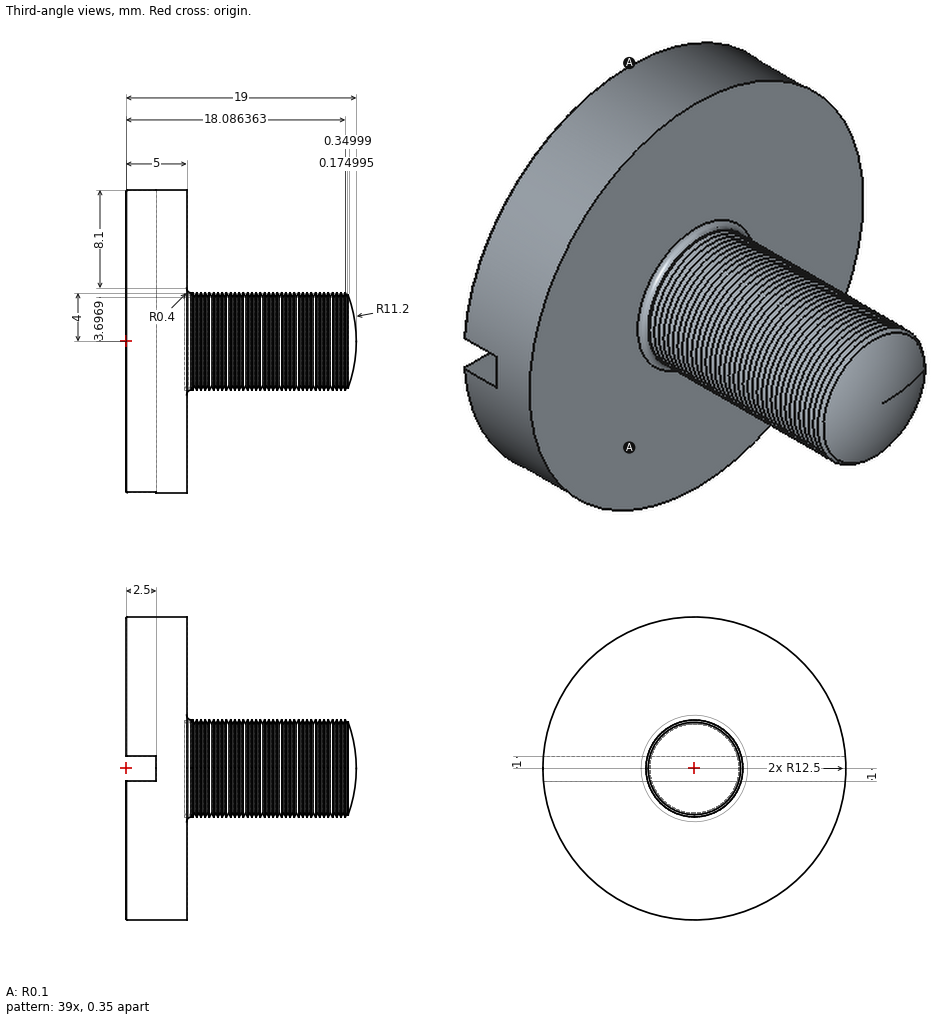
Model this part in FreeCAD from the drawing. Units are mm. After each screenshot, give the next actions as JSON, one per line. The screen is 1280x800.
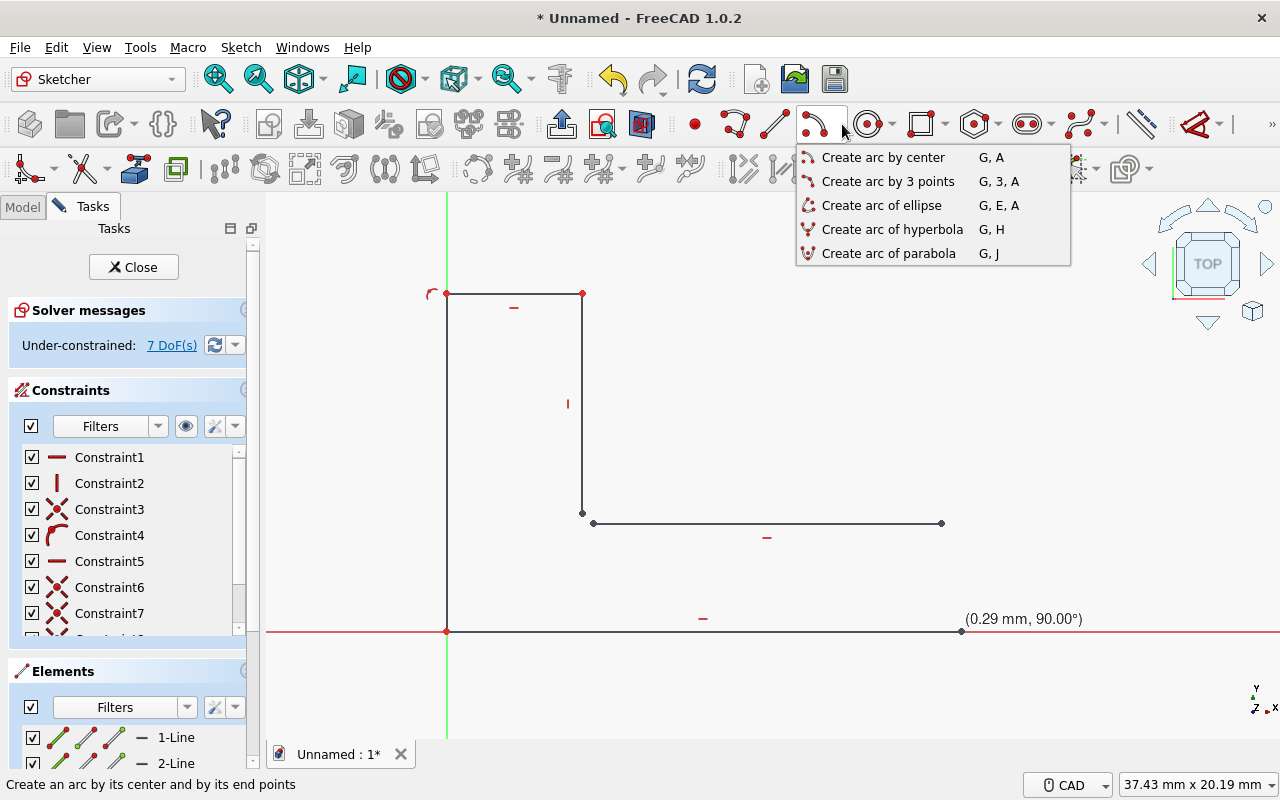
{"action": "left_click", "coordinate": [934, 181]}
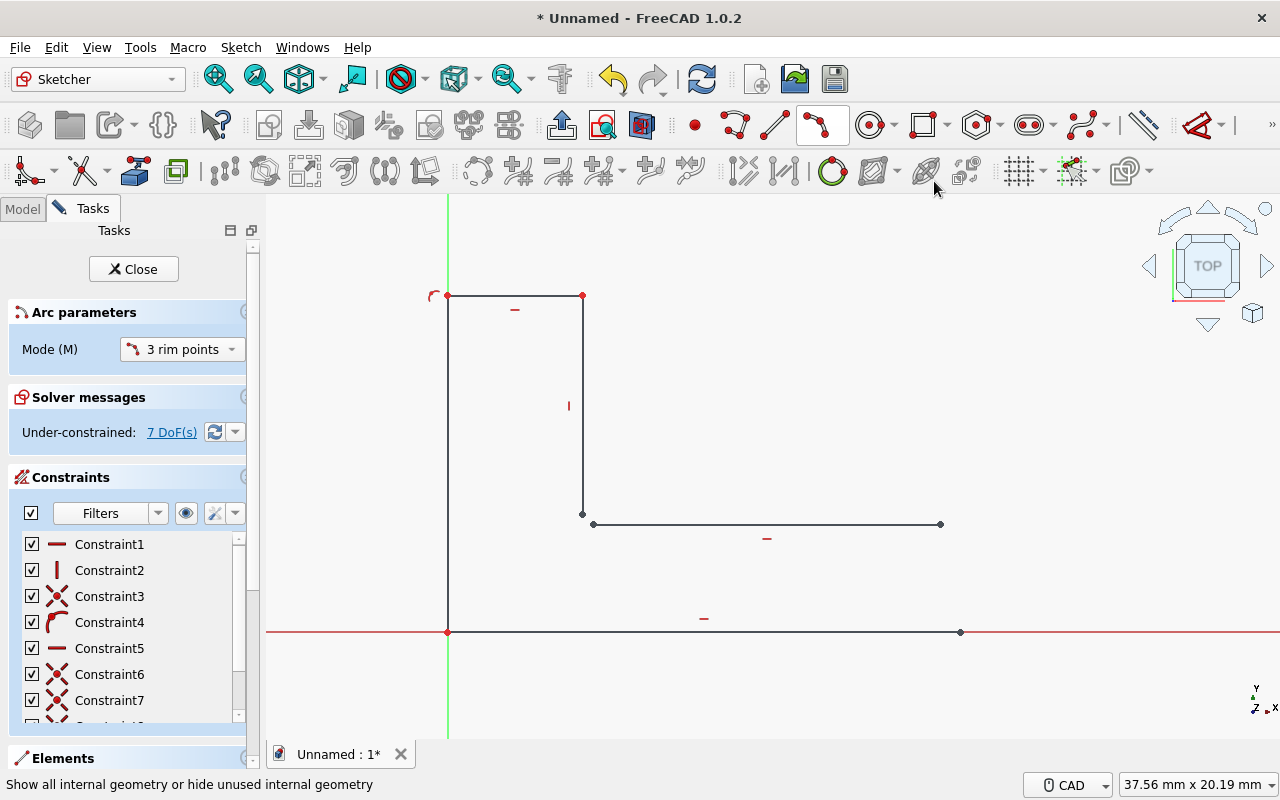
{"action": "left_click", "coordinate": [594, 525]}
{"action": "left_click", "coordinate": [583, 515]}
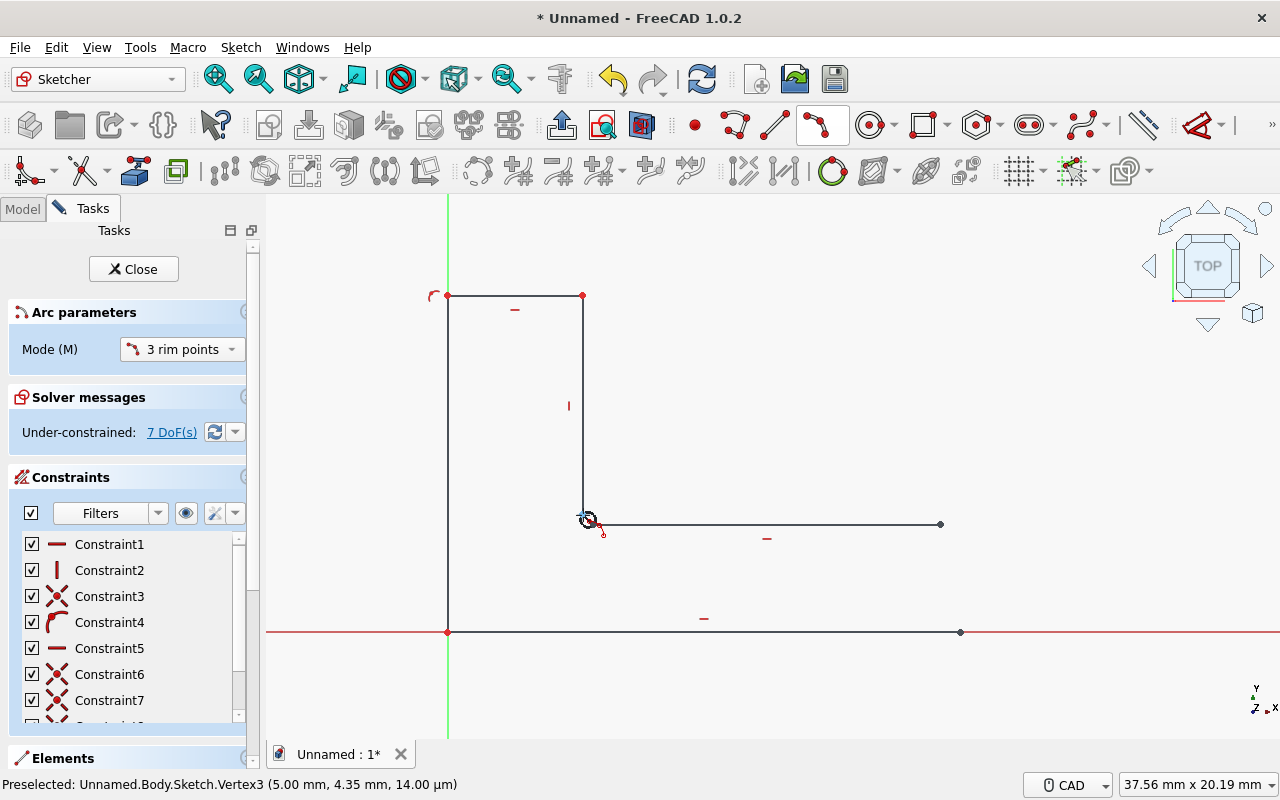
{"action": "scroll", "coordinate": [586, 521], "scroll_direction": "up", "scroll_amount": 9}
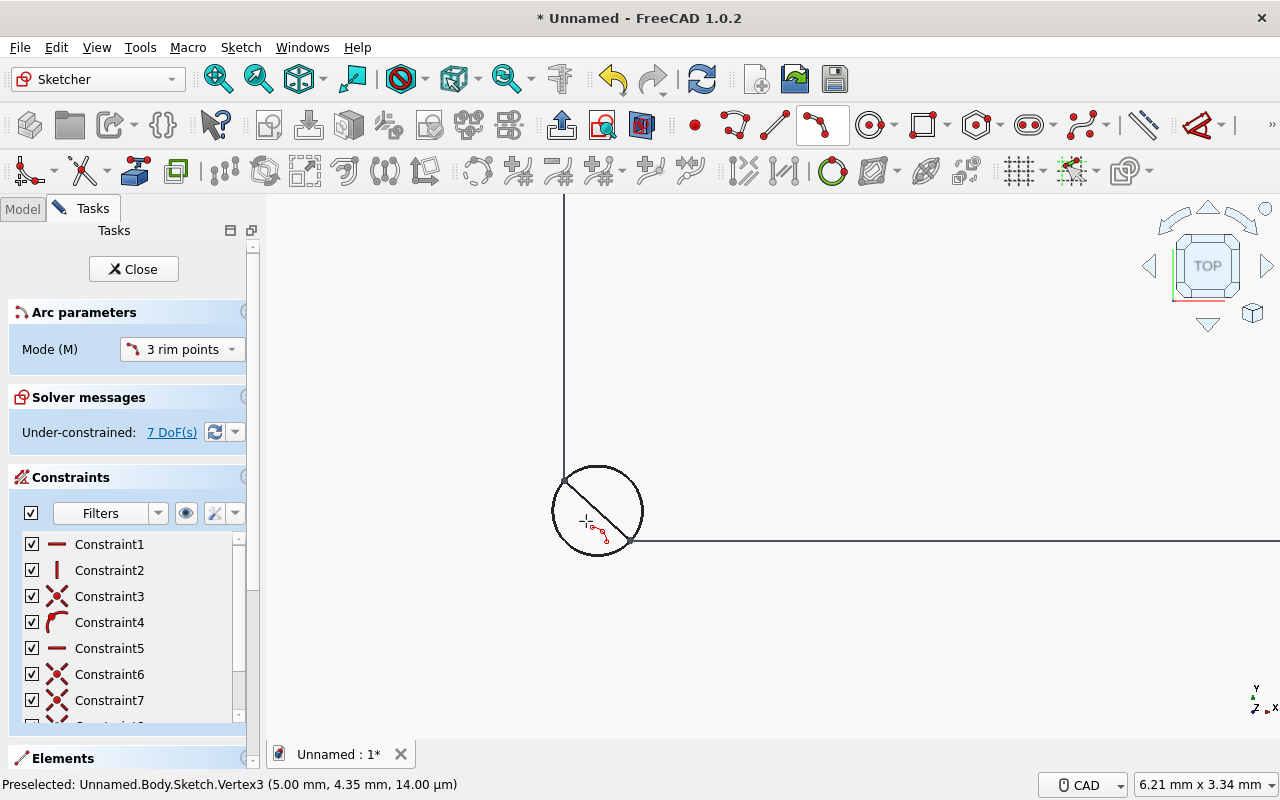
{"action": "left_click", "coordinate": [584, 518]}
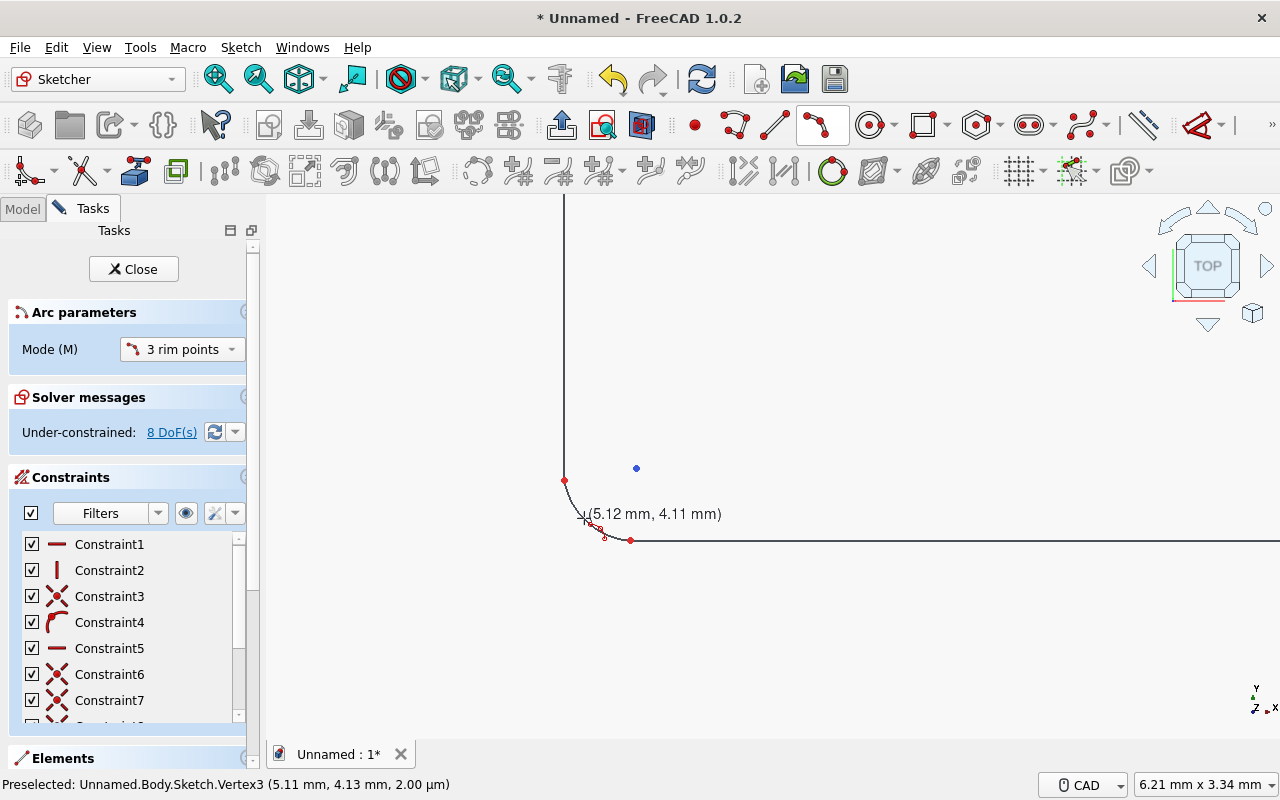
{"action": "scroll", "coordinate": [587, 525], "scroll_direction": "down", "scroll_amount": 9}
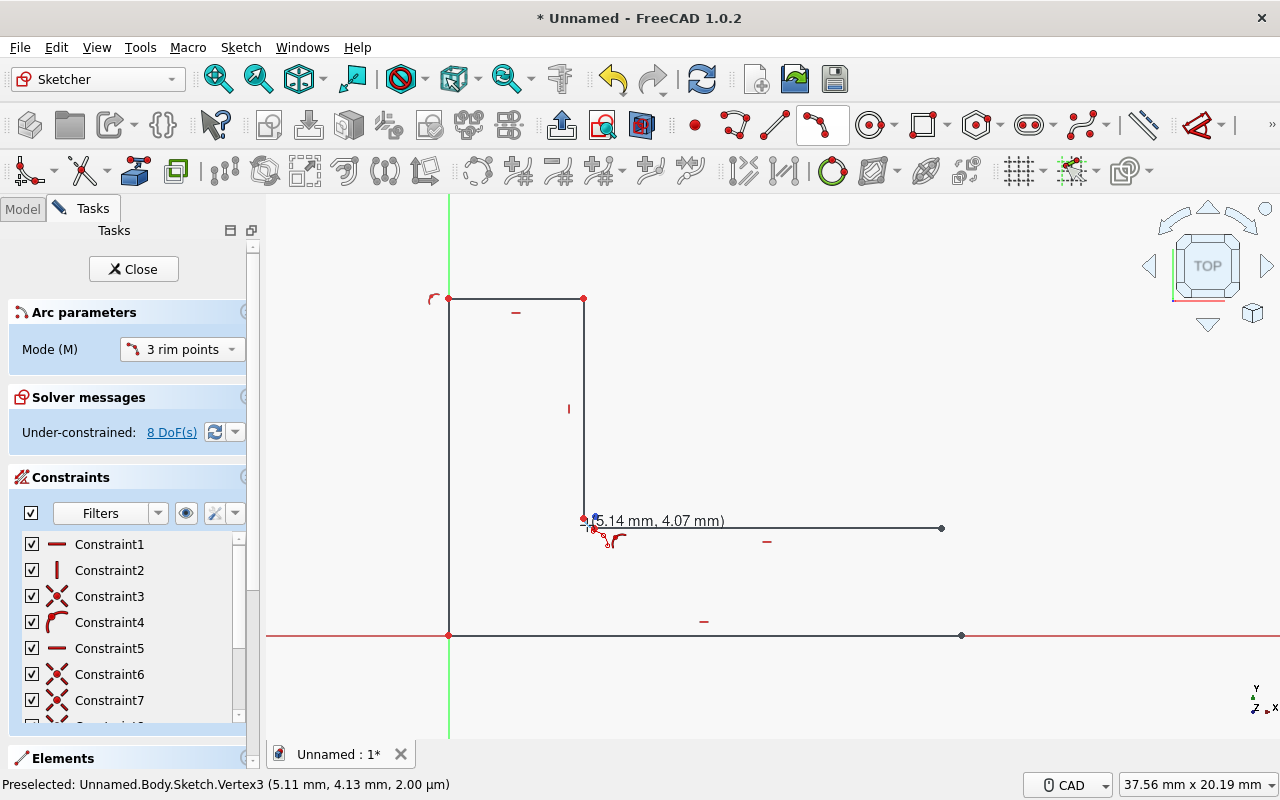
{"action": "left_click", "coordinate": [961, 636]}
{"action": "left_click", "coordinate": [941, 528]}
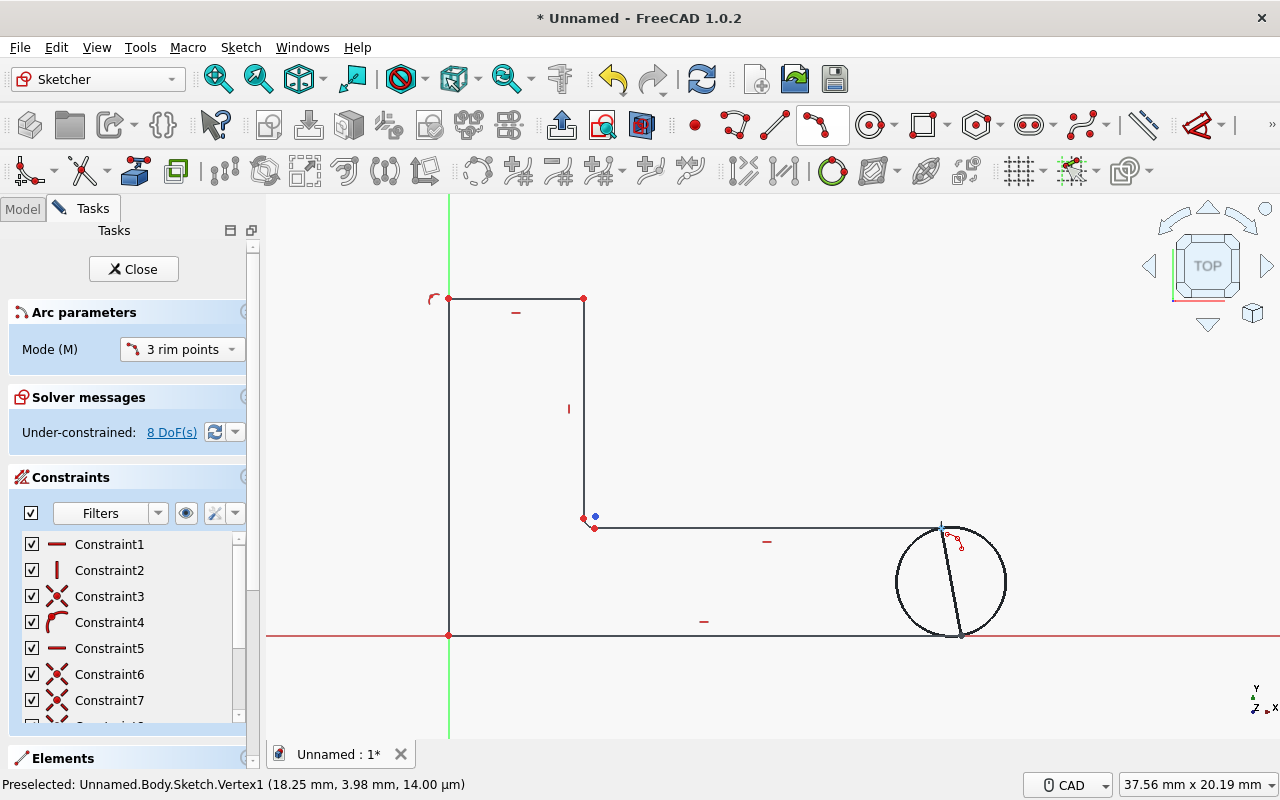
{"action": "scroll", "coordinate": [956, 581], "scroll_direction": "up", "scroll_amount": 6}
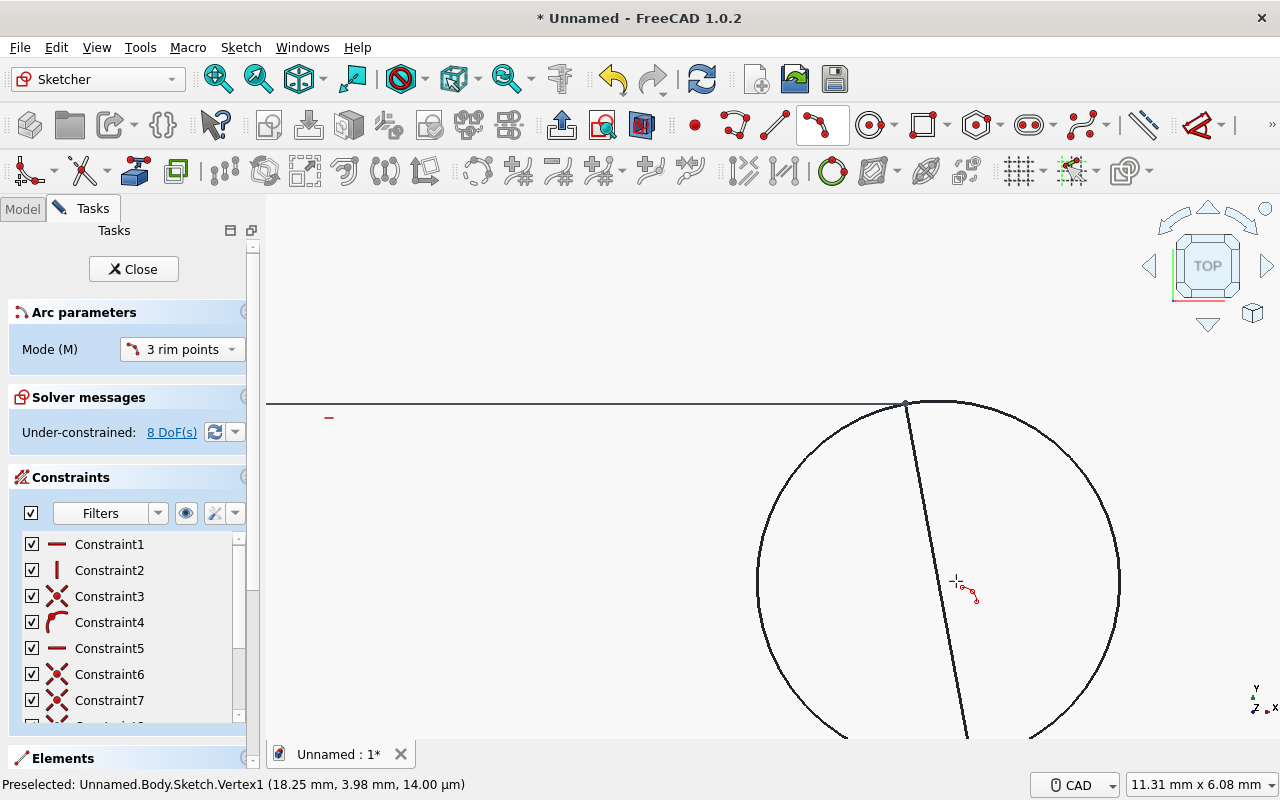
{"action": "left_click", "coordinate": [956, 578]}
{"action": "key", "text": "Escape"}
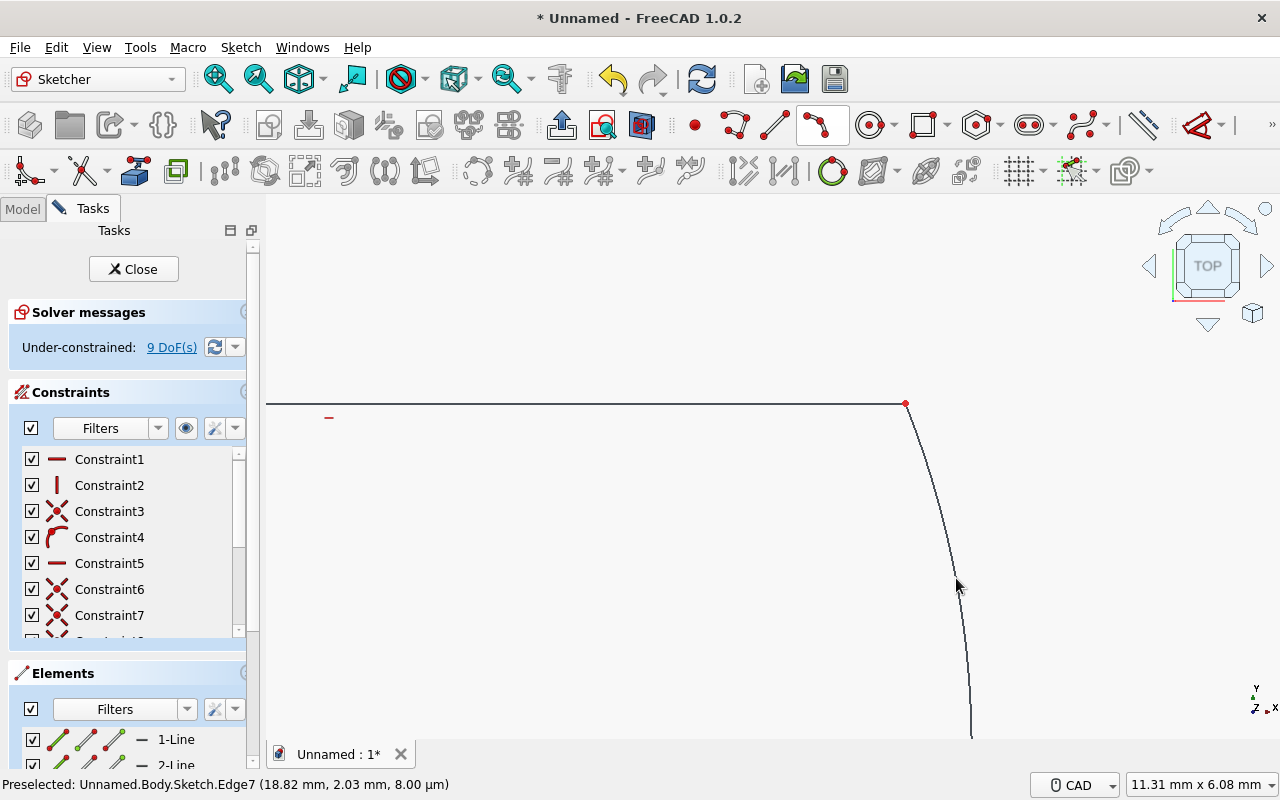
{"action": "left_click", "coordinate": [560, 404]}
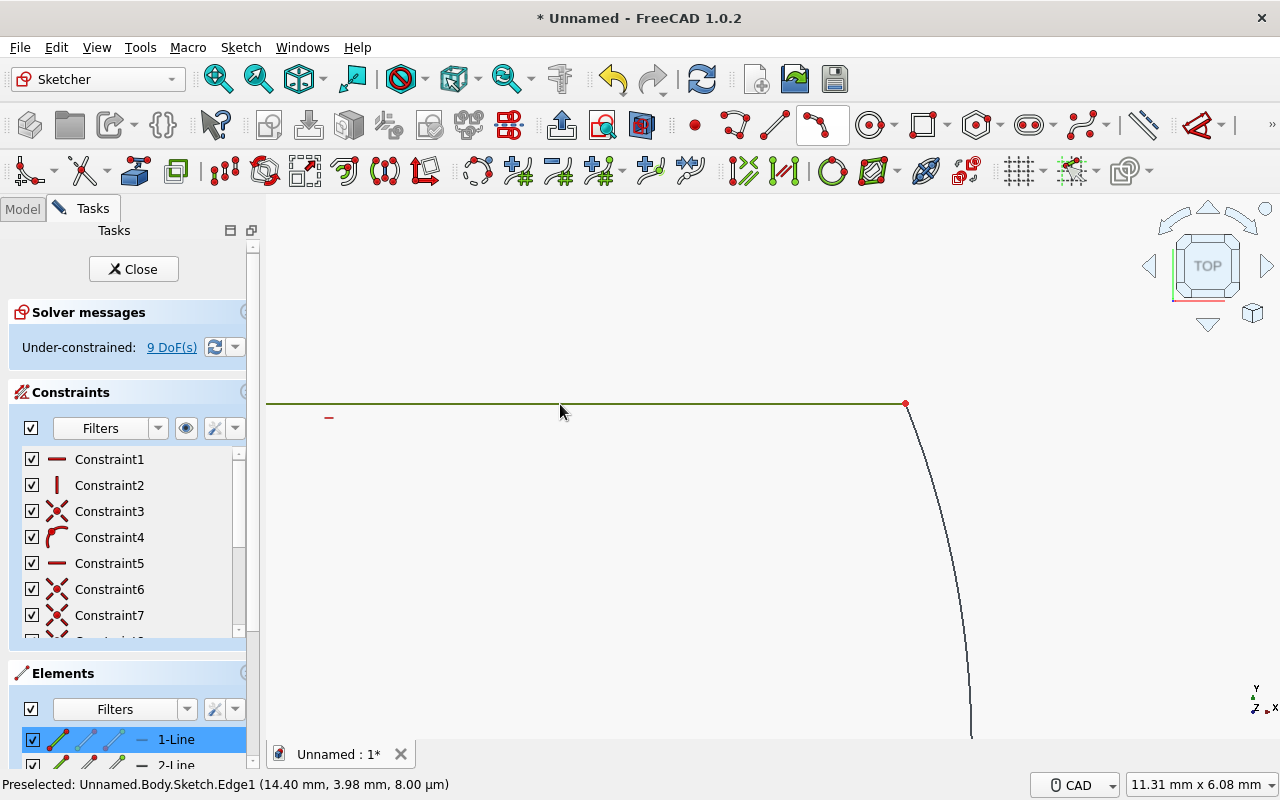
{"action": "scroll", "coordinate": [956, 581], "scroll_direction": "down", "scroll_amount": 6}